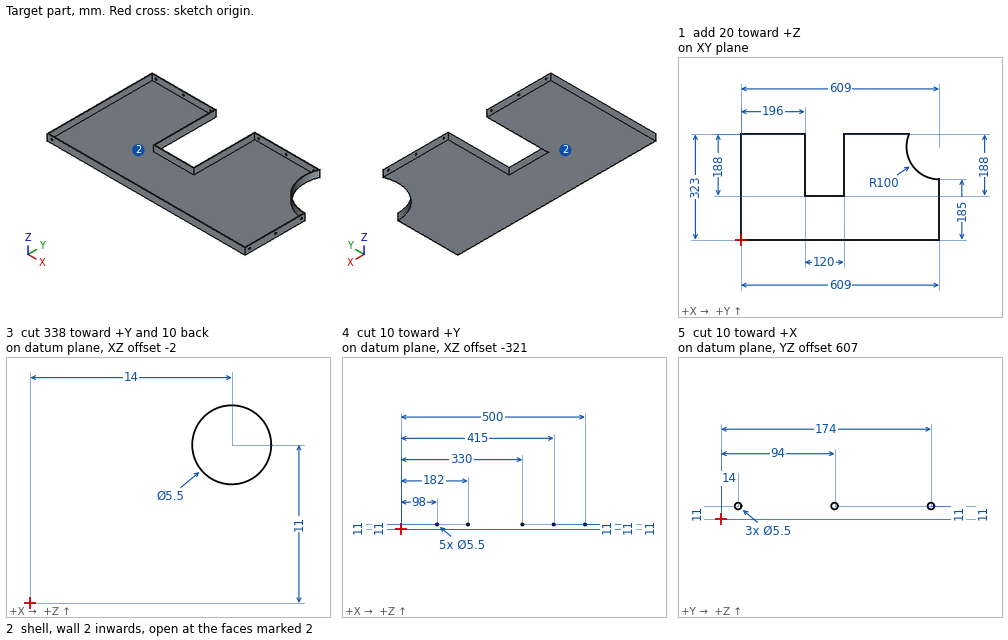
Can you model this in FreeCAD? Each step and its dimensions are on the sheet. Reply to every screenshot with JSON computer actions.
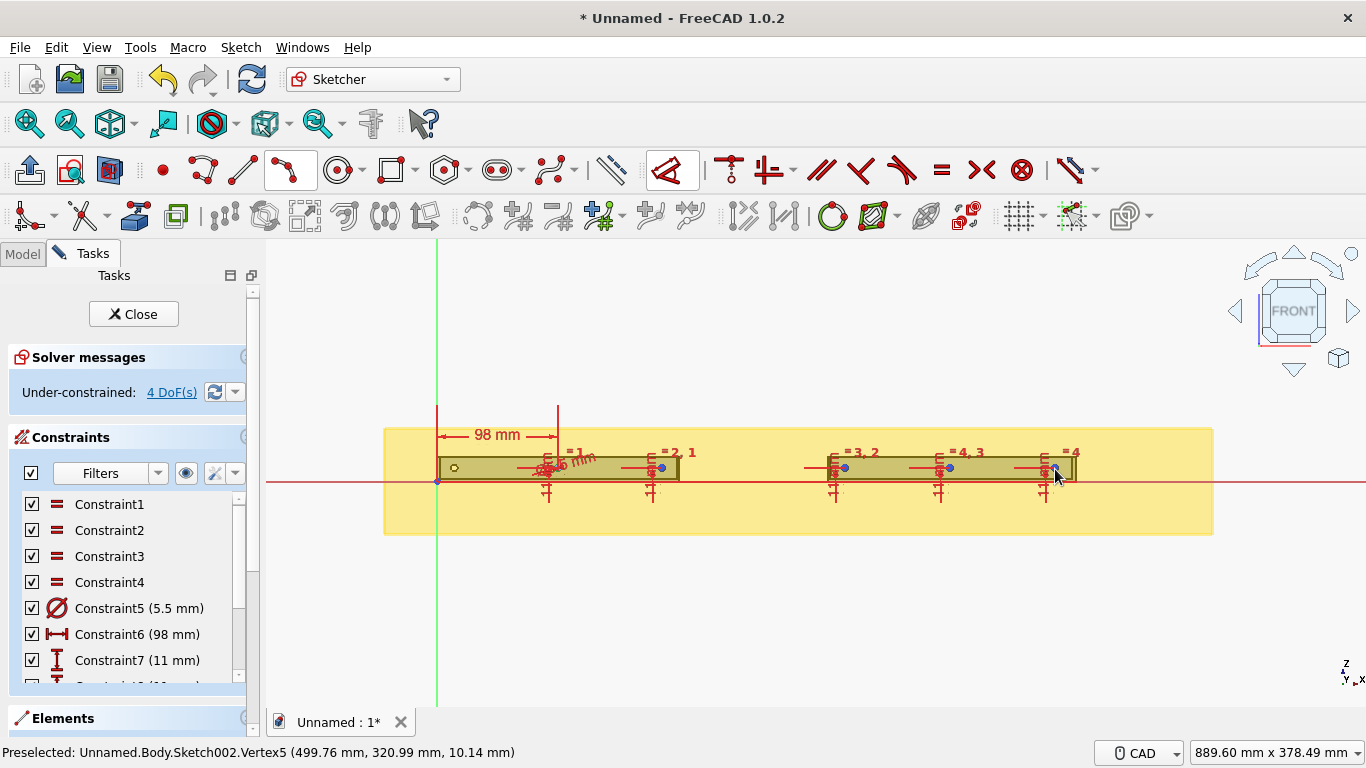
{"action": "left_click", "coordinate": [662, 468]}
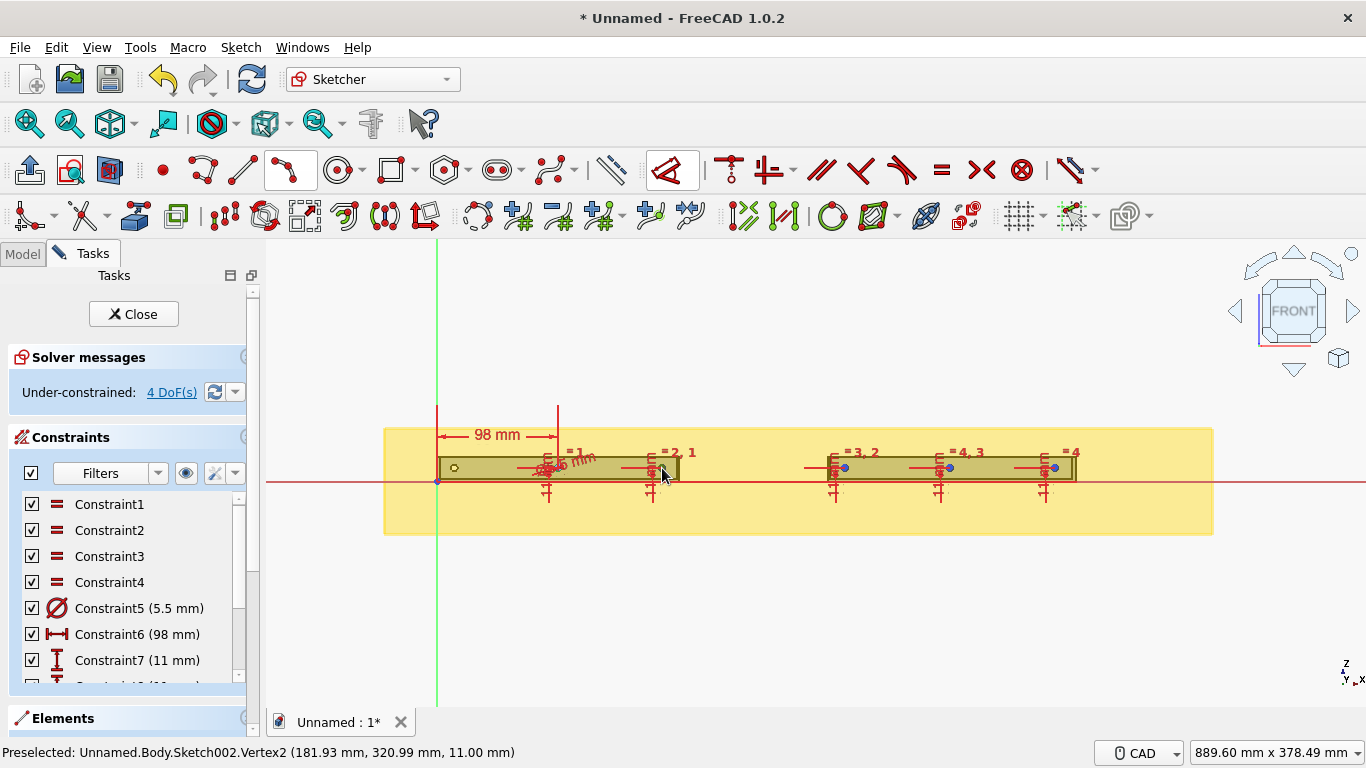
{"action": "left_click", "coordinate": [694, 170]}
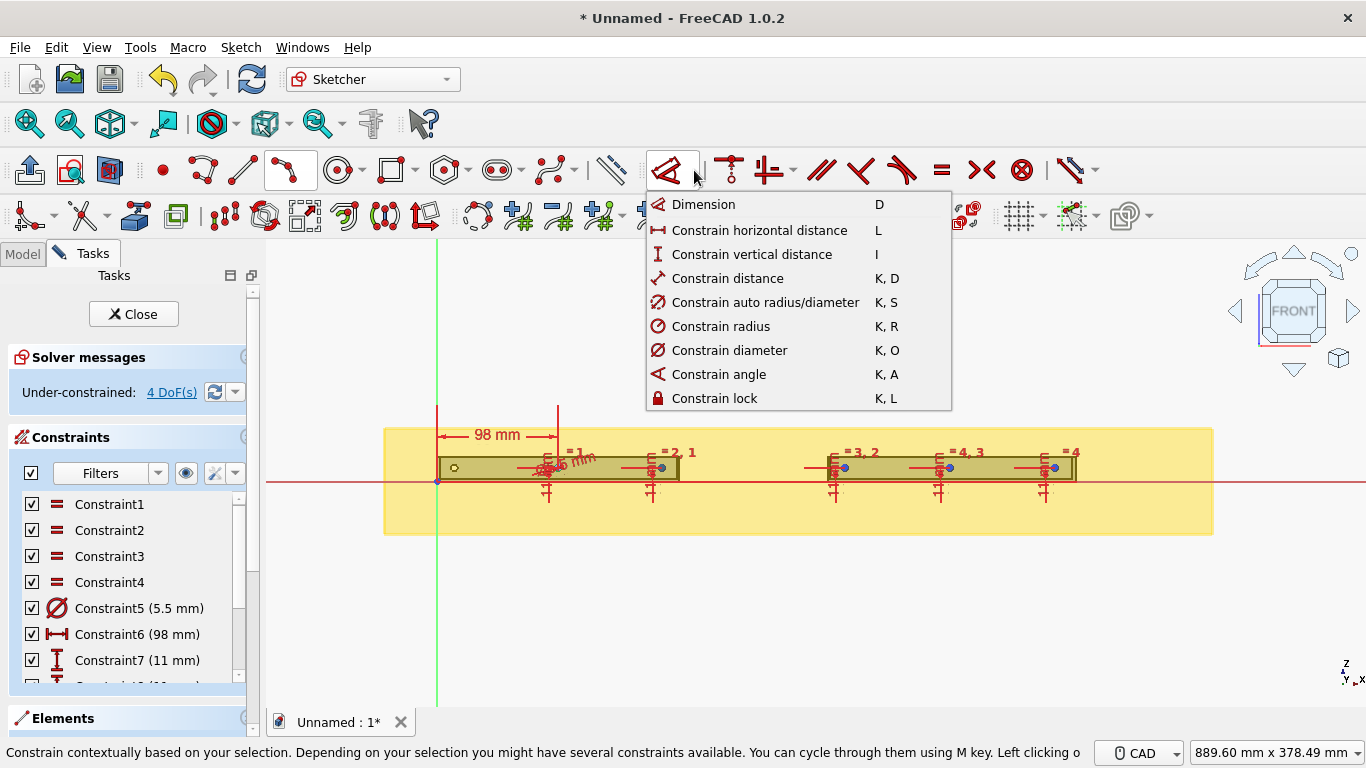
{"action": "left_click", "coordinate": [799, 230]}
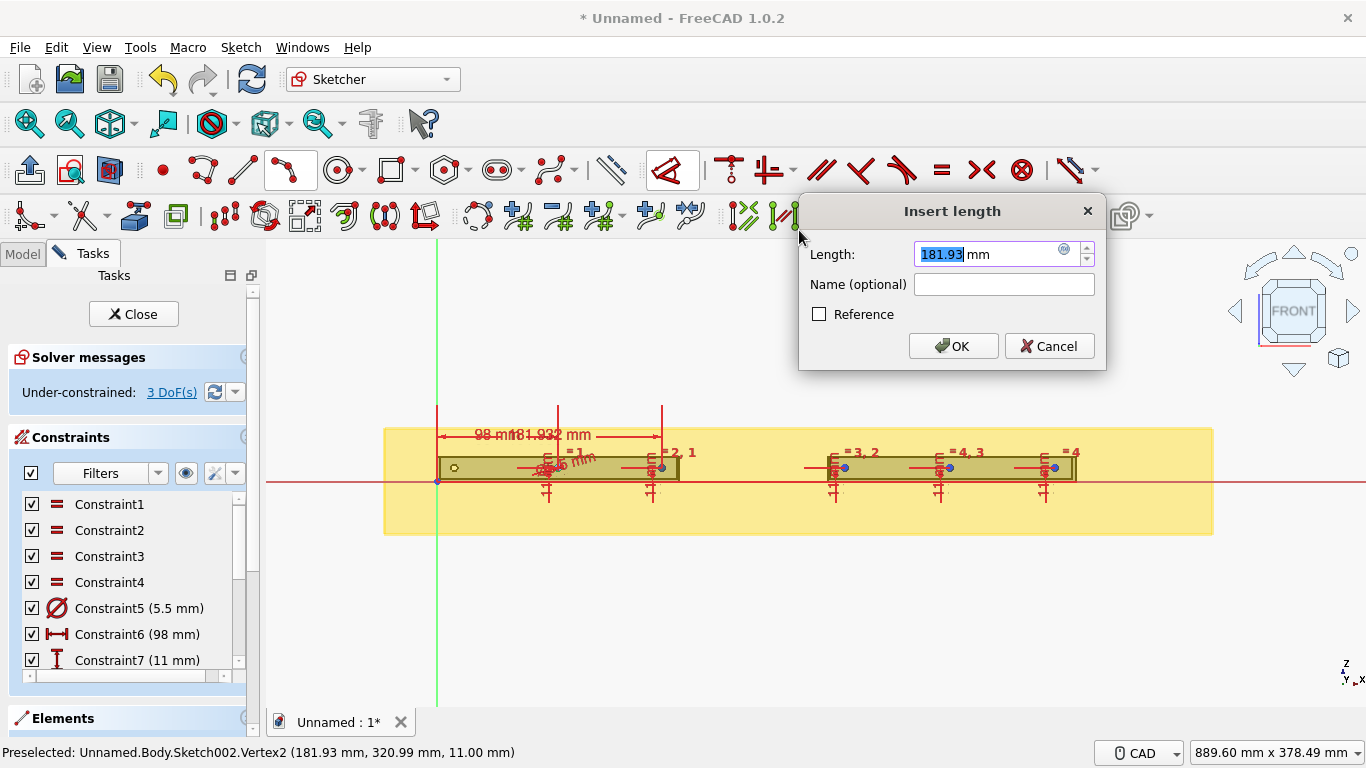
{"action": "type", "text": "182"}
{"action": "key", "text": "Return"}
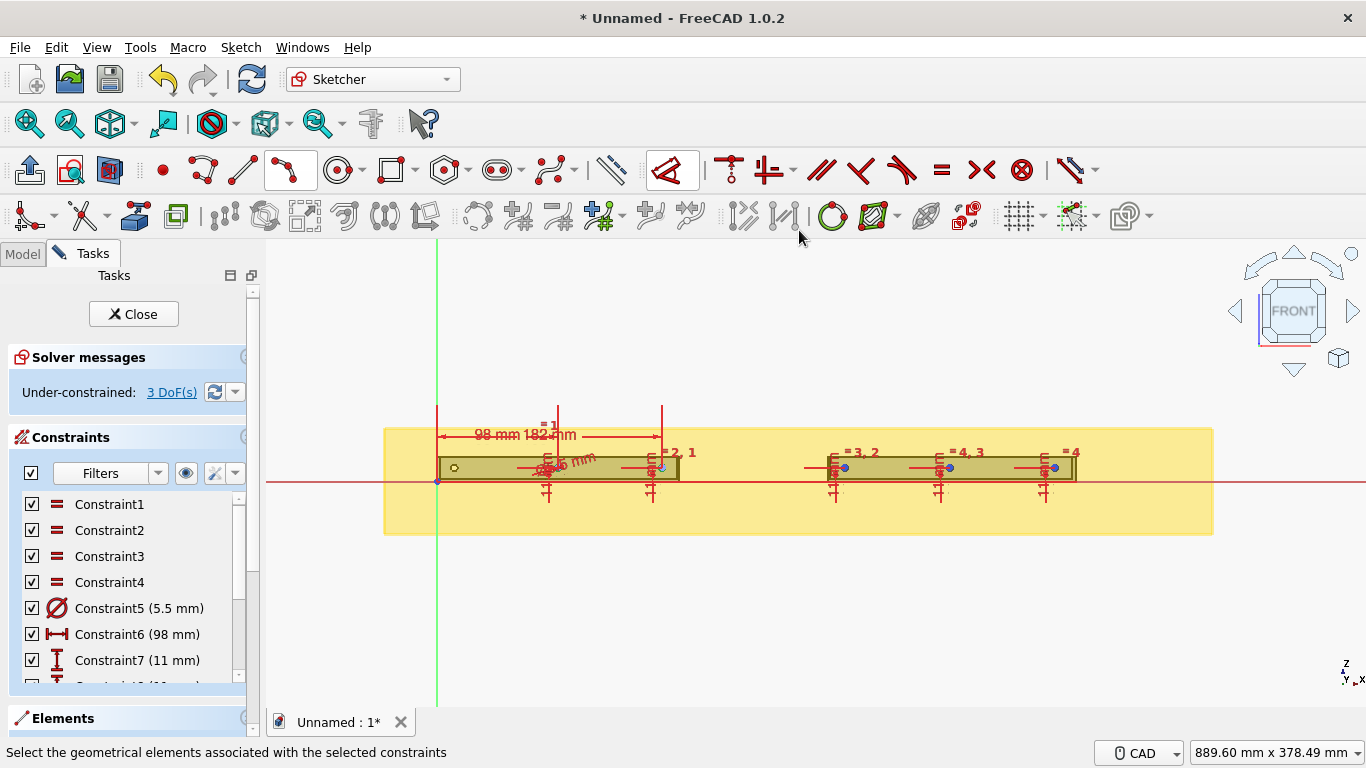
{"action": "left_click", "coordinate": [845, 468]}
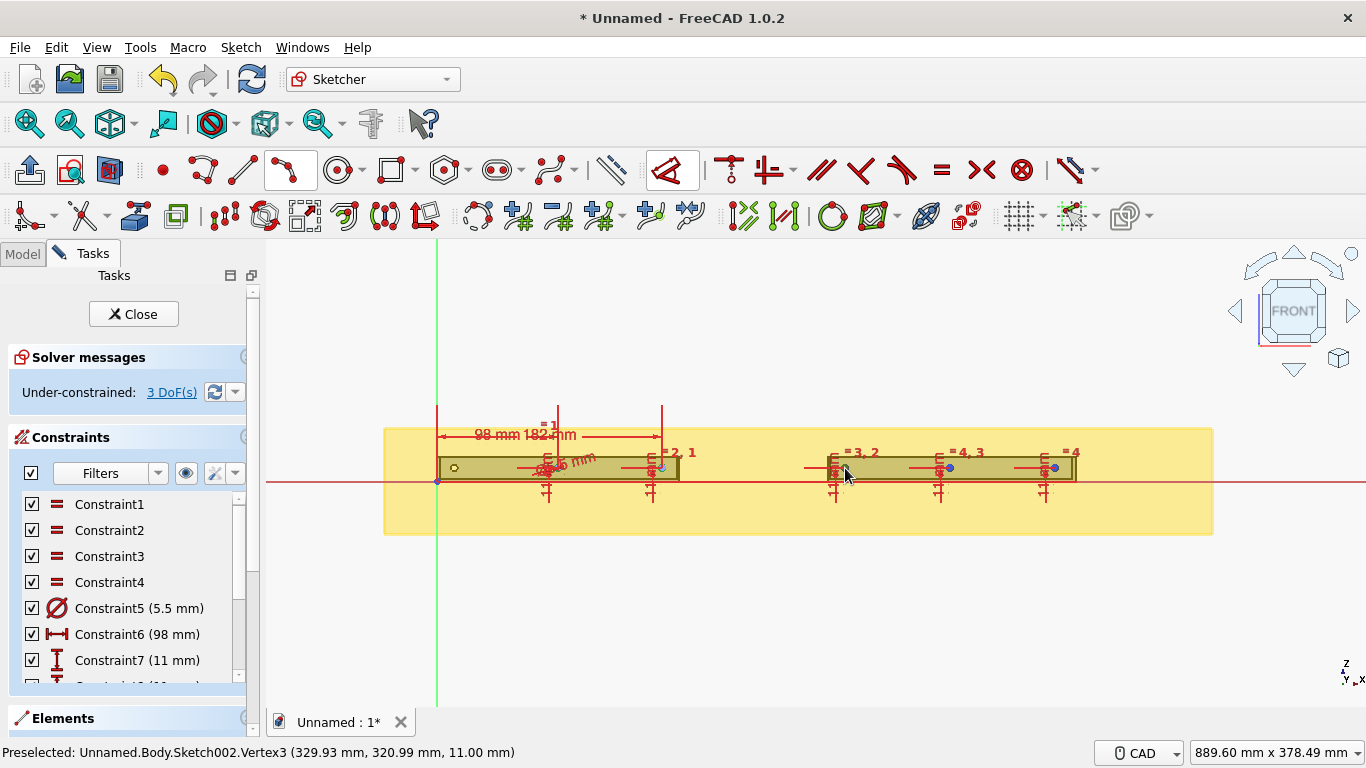
{"action": "key", "text": "l"}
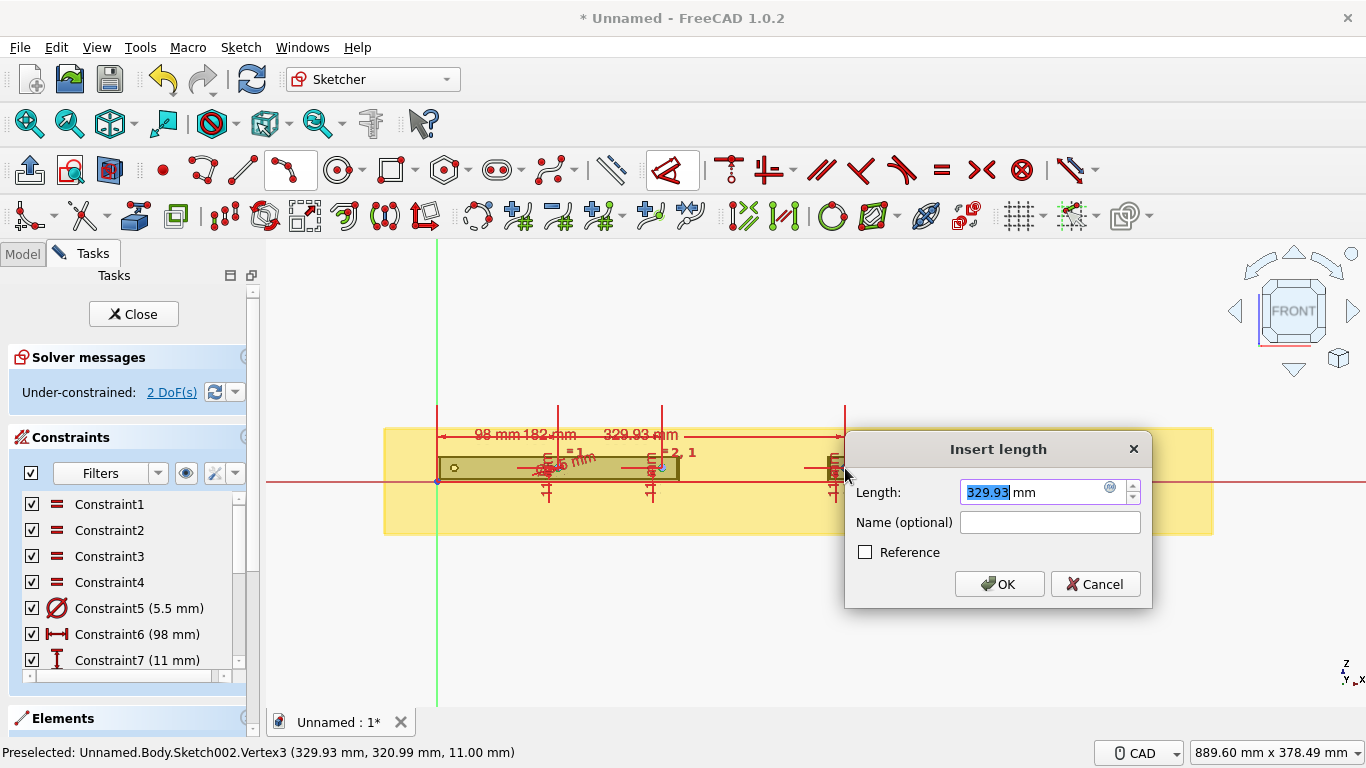
{"action": "type", "text": "330"}
{"action": "key", "text": "Return"}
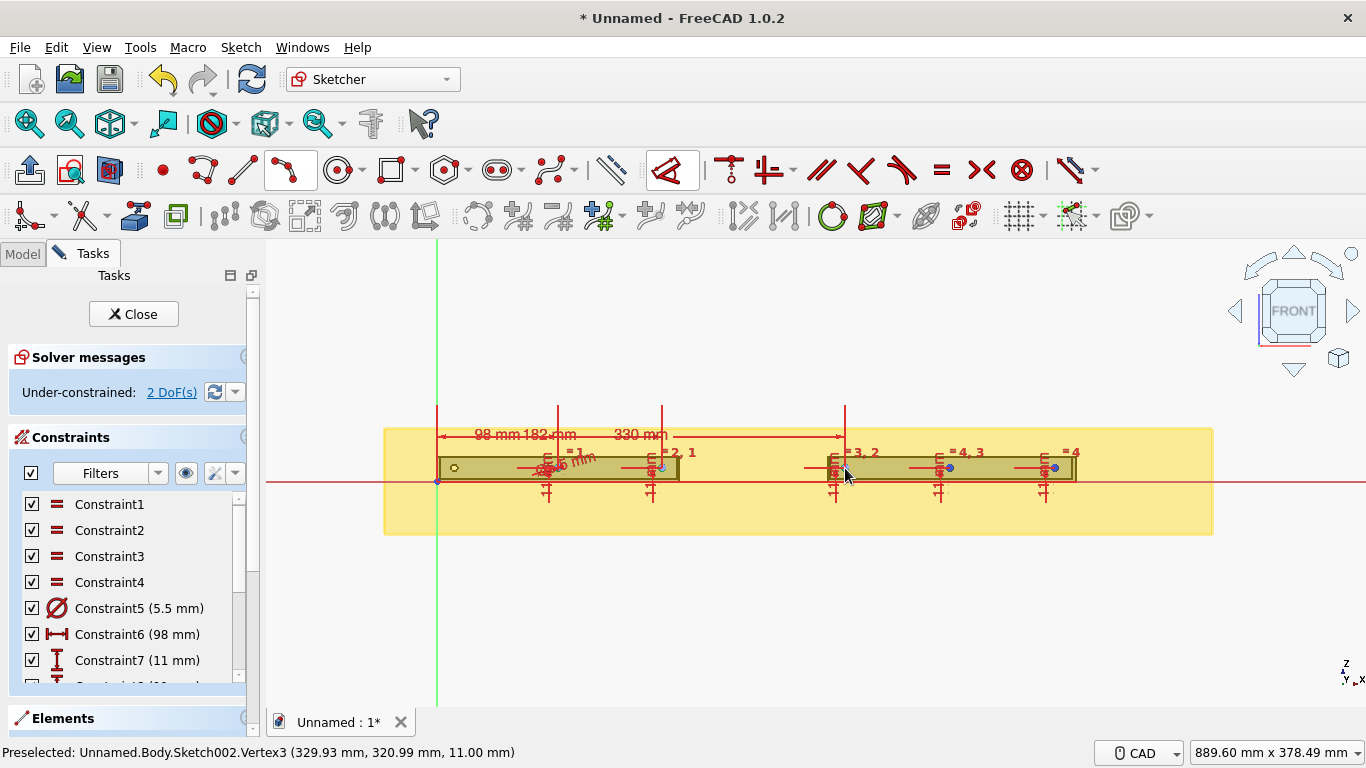
{"action": "left_click", "coordinate": [950, 468]}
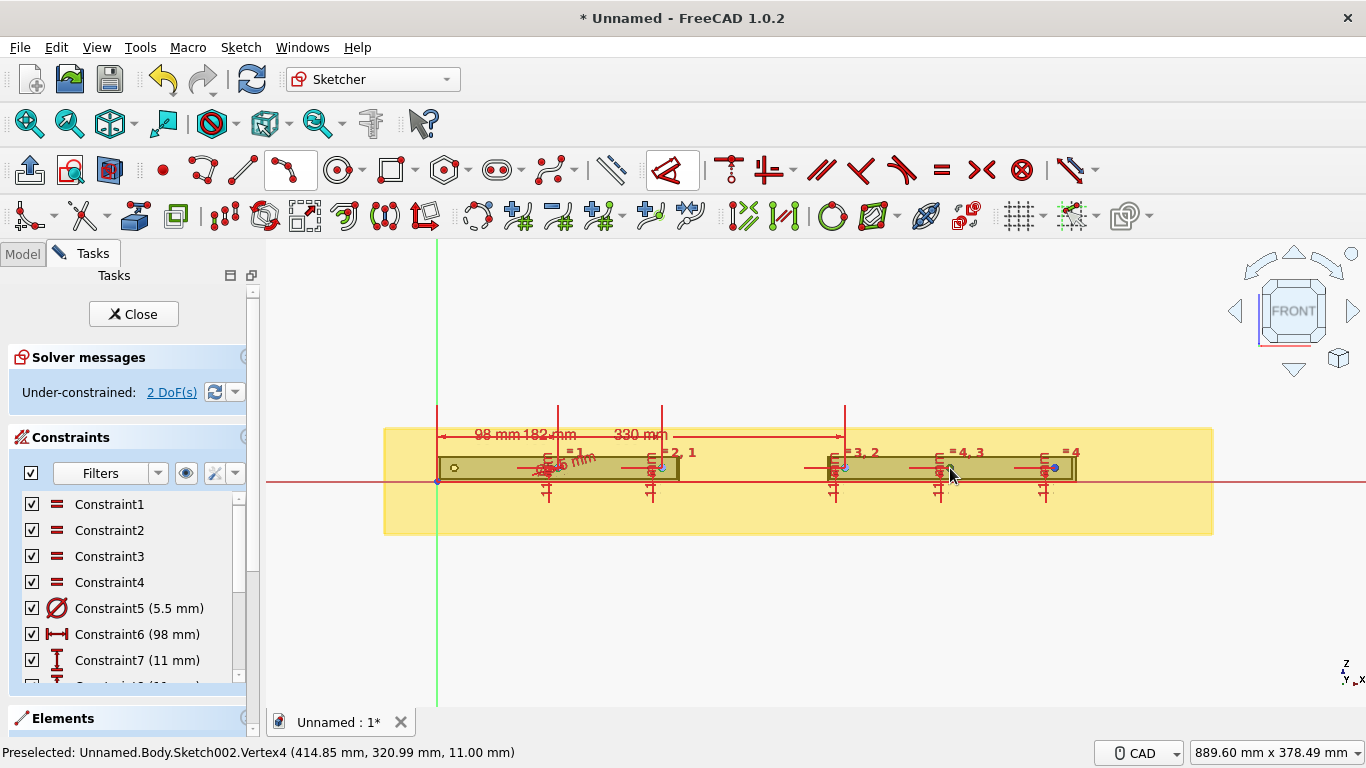
{"action": "key", "text": "l"}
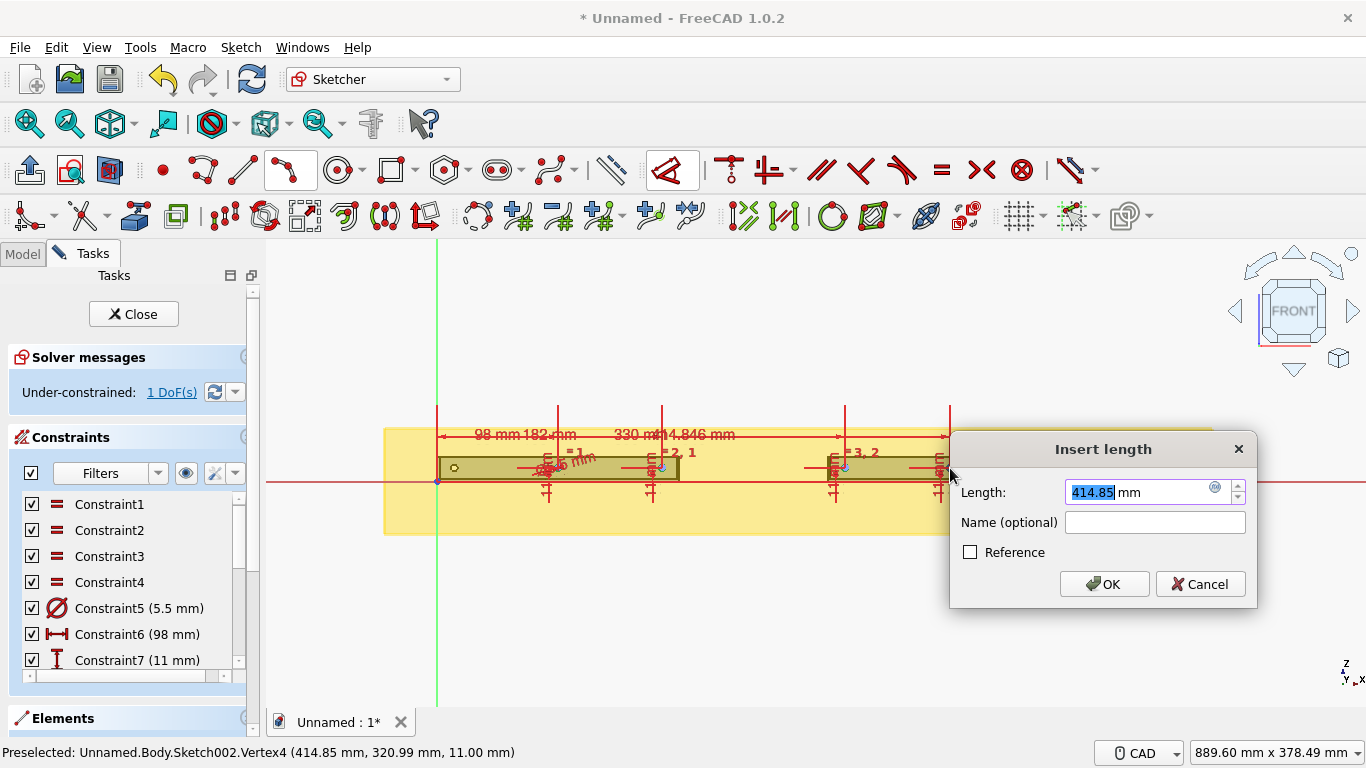
{"action": "type", "text": "415"}
{"action": "key", "text": "Return"}